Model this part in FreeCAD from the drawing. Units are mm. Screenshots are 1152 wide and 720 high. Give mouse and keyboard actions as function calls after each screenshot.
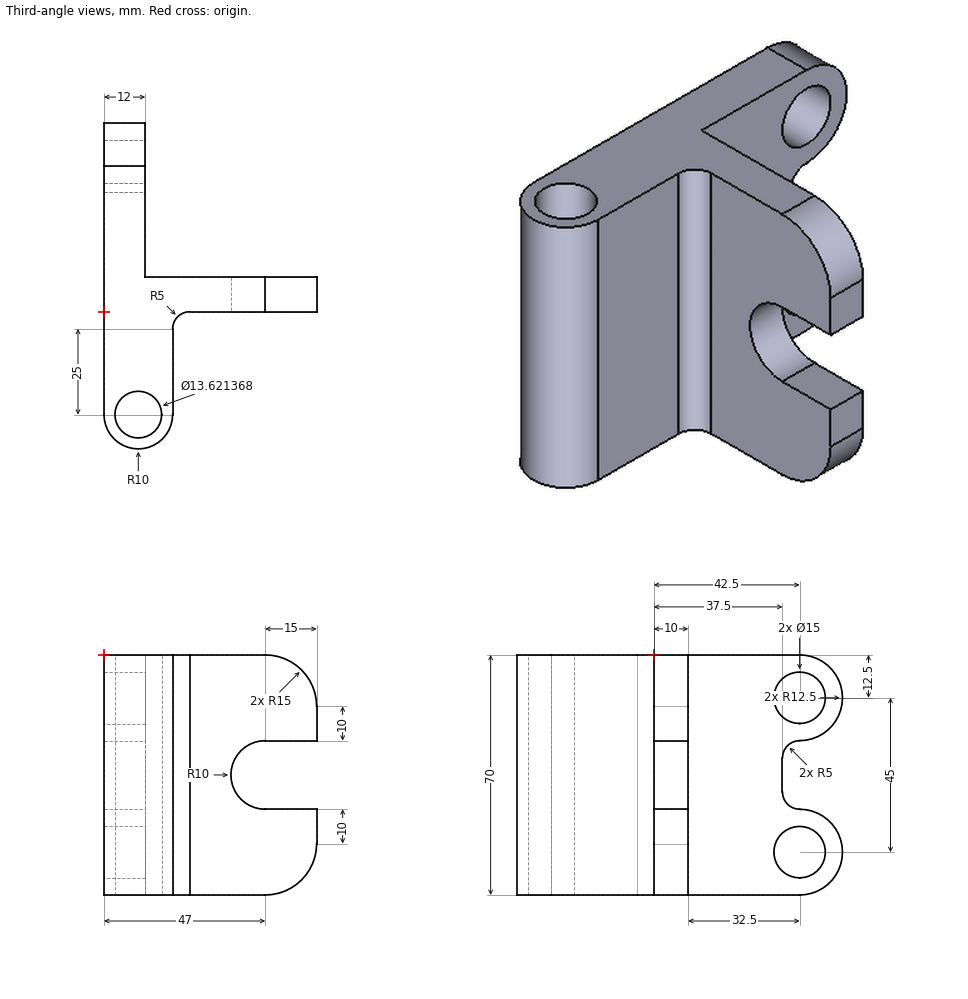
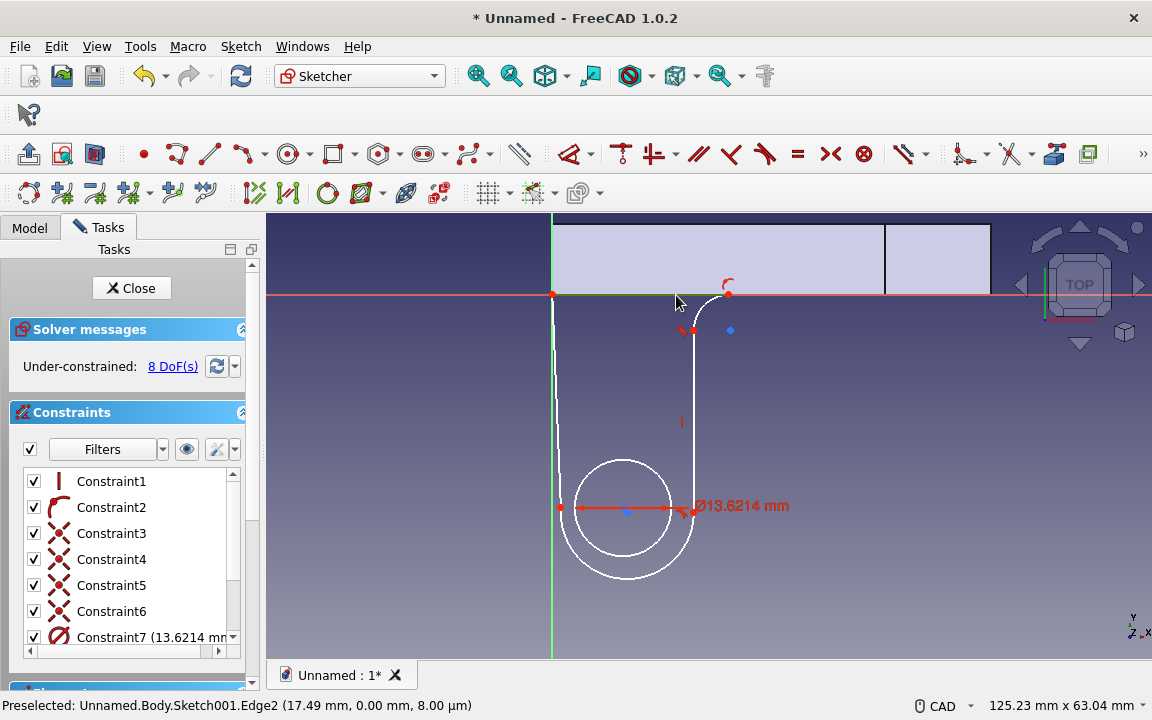
click(698, 315)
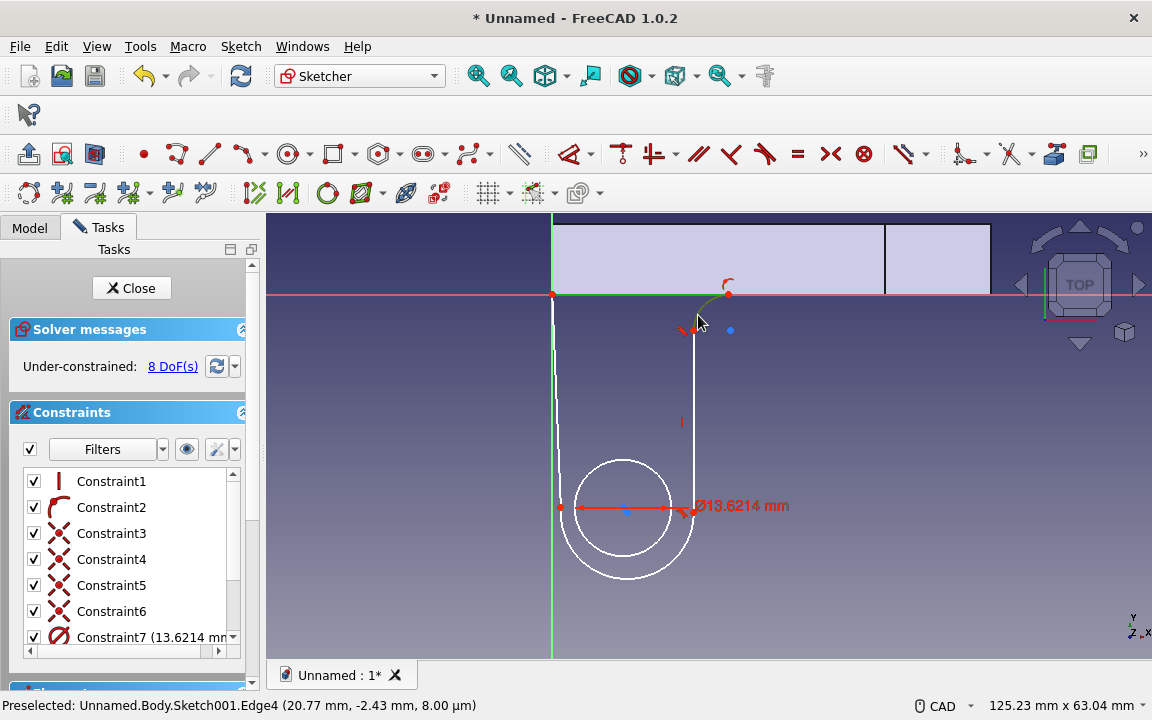
click(765, 154)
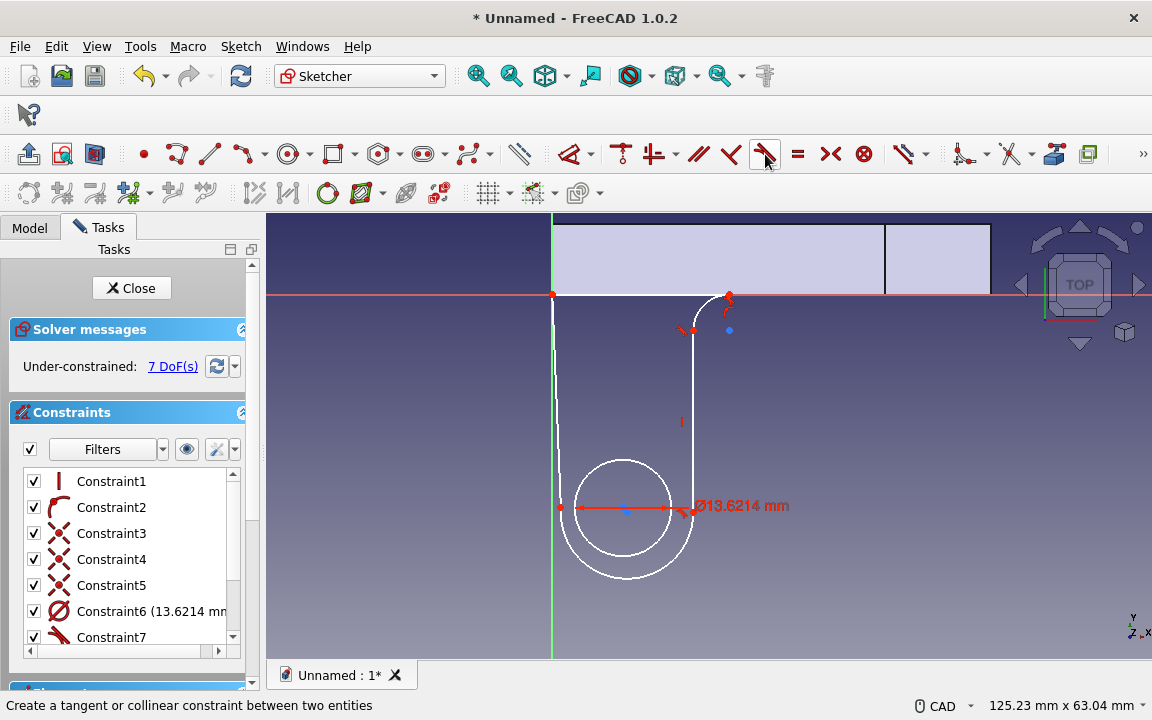
click(555, 359)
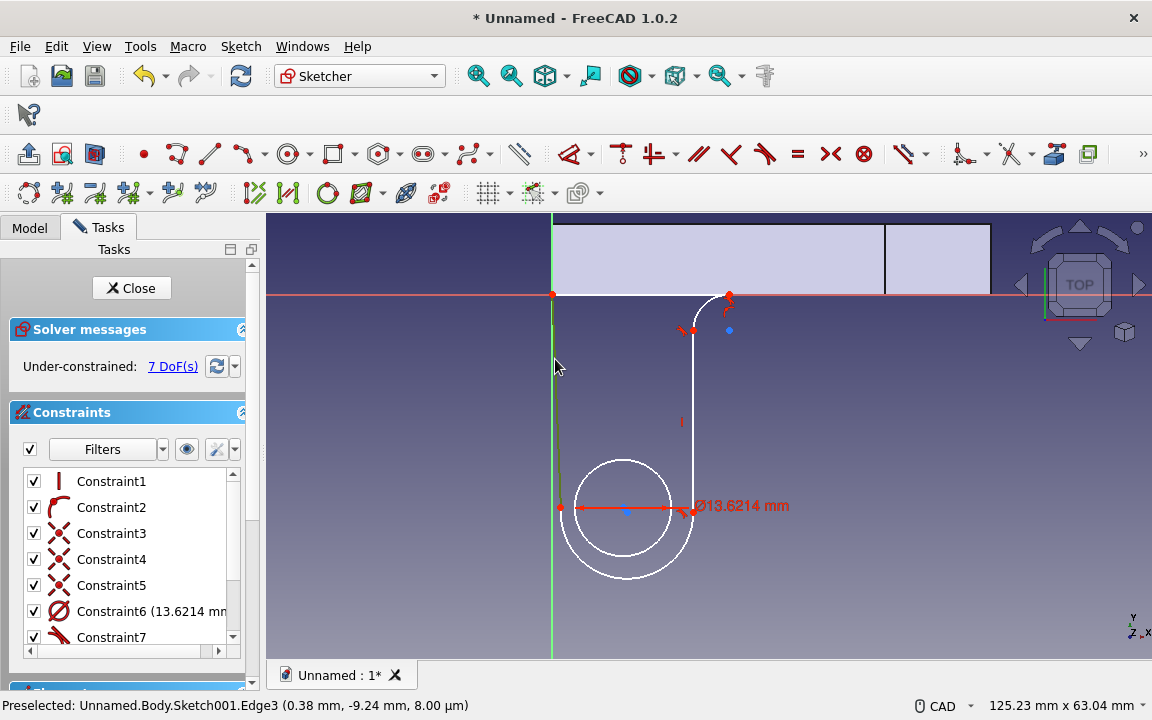
click(586, 564)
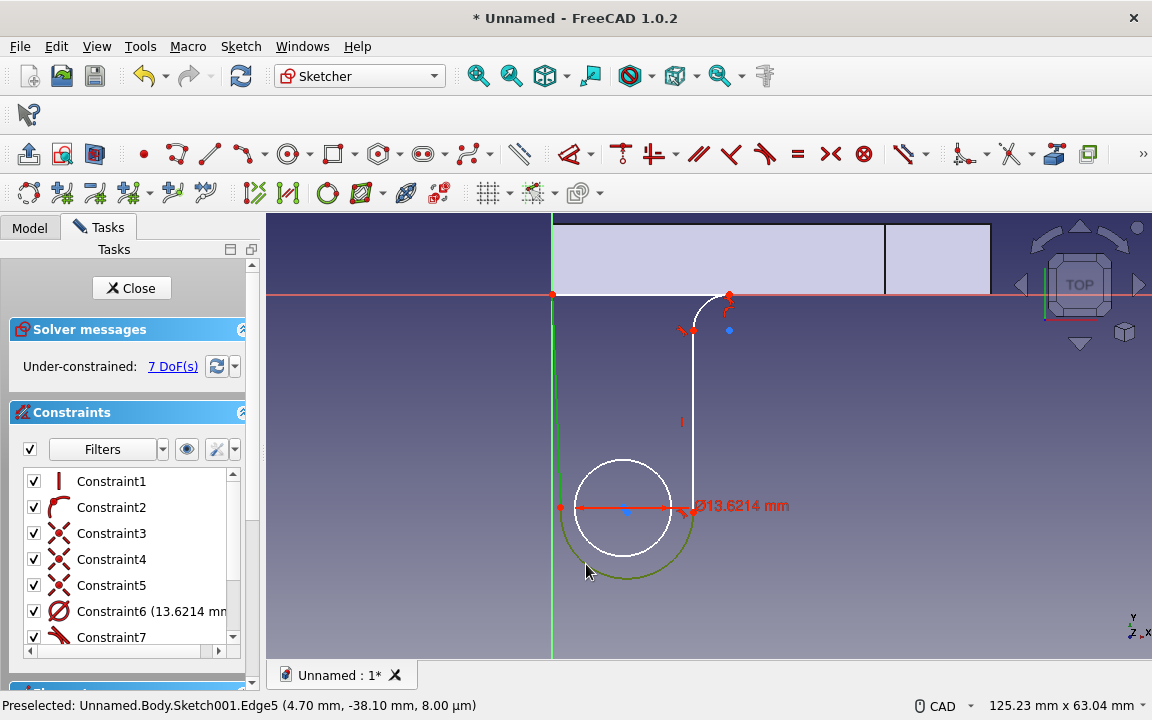
key(t)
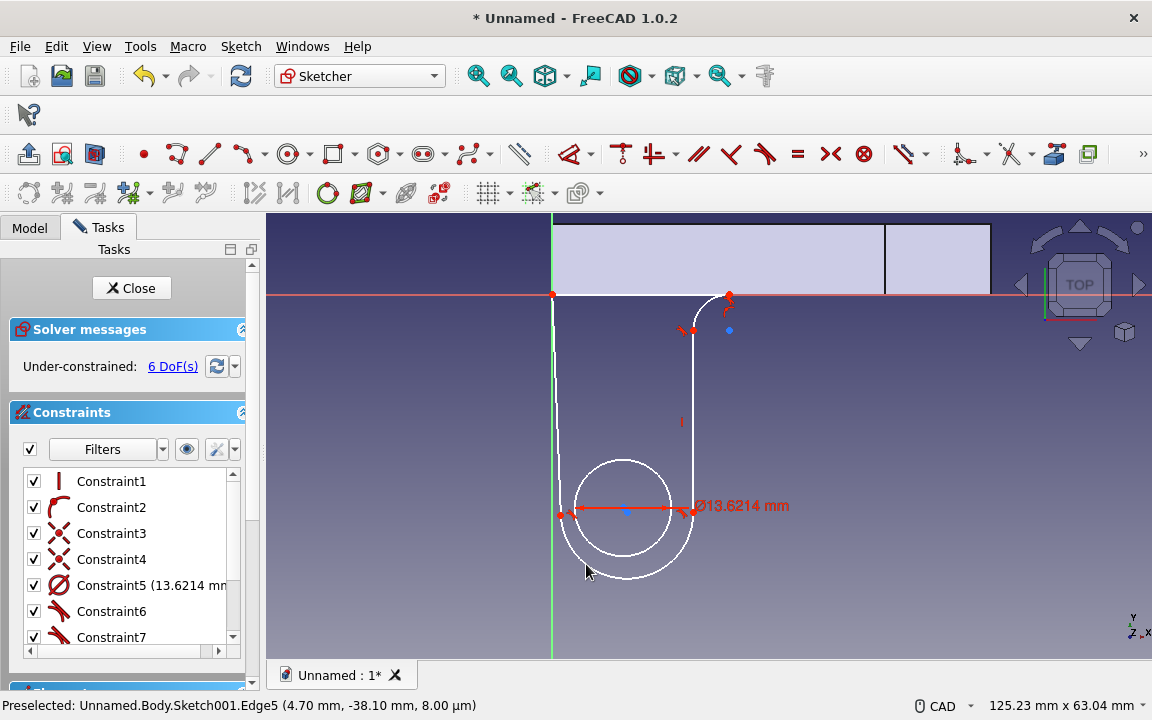
click(555, 361)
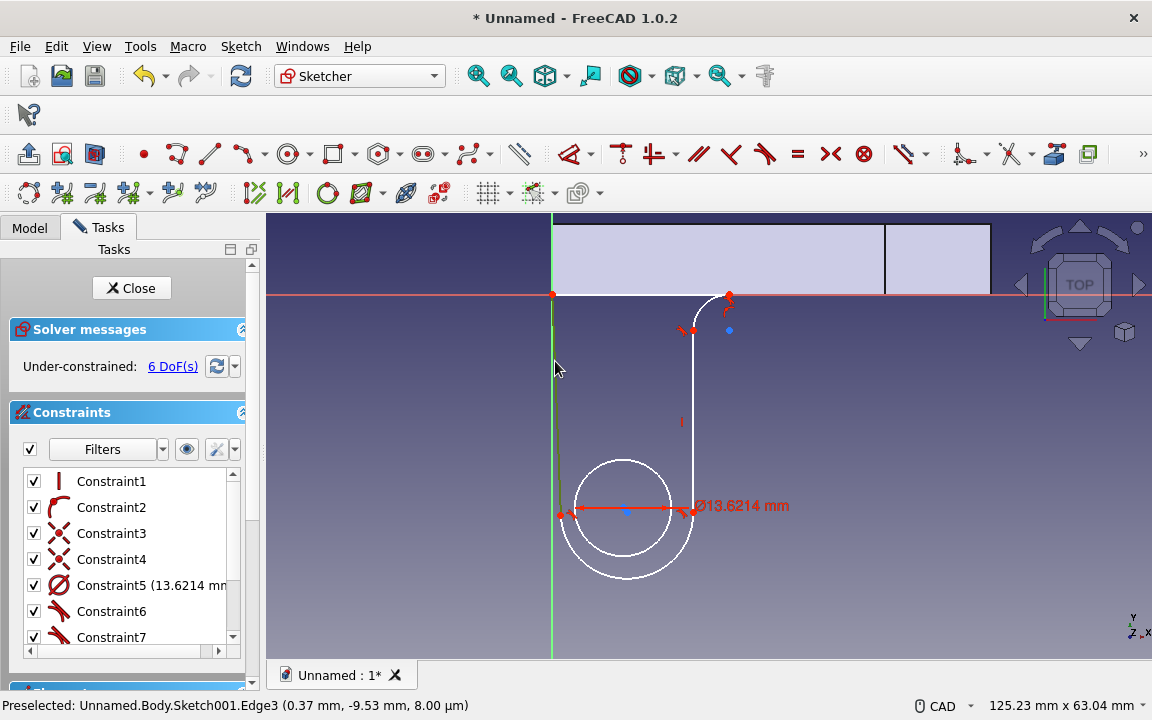
key(v)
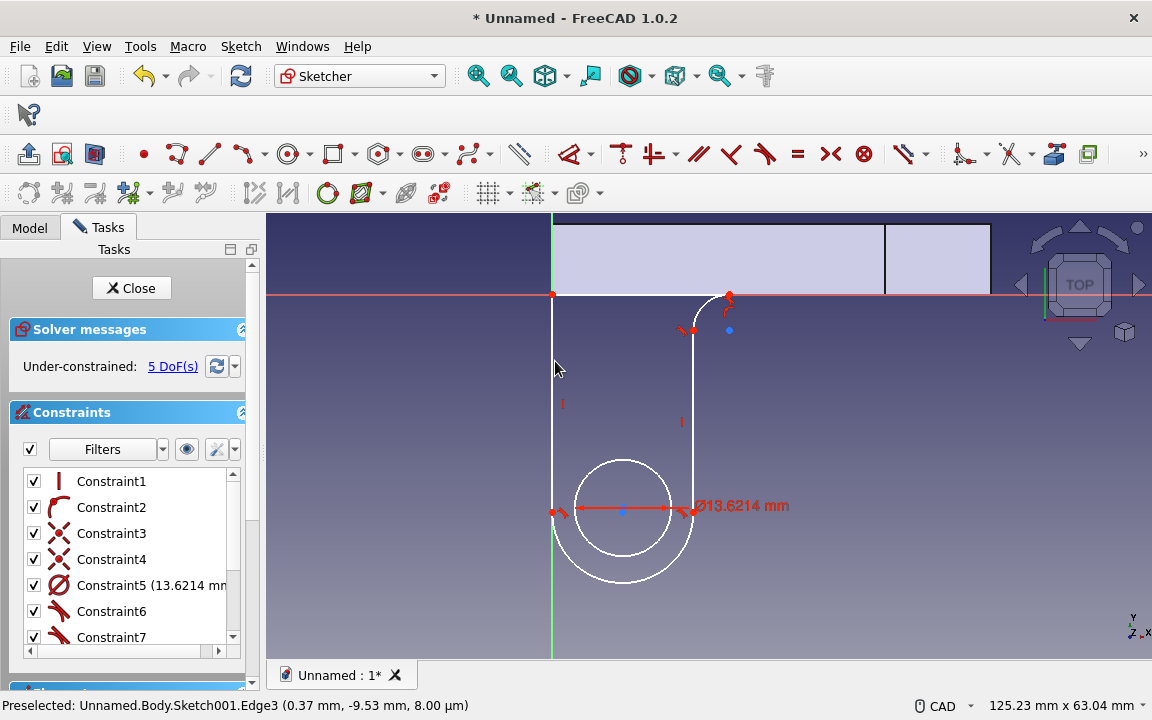
click(657, 474)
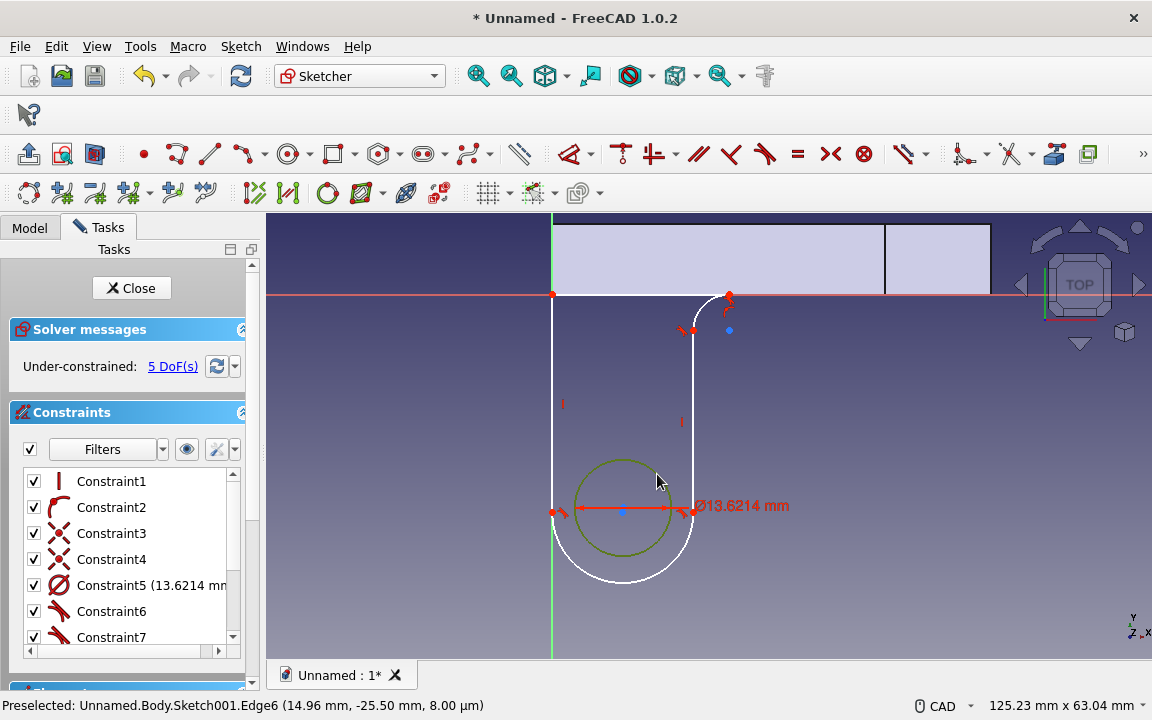
click(581, 570)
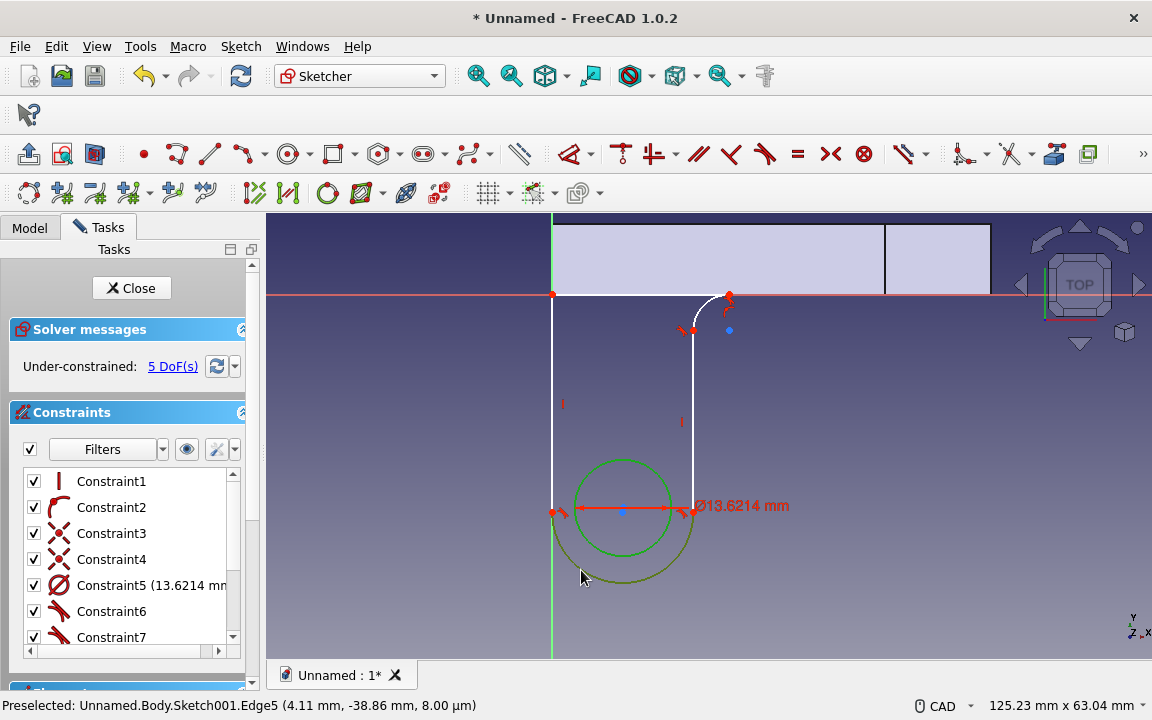
click(621, 154)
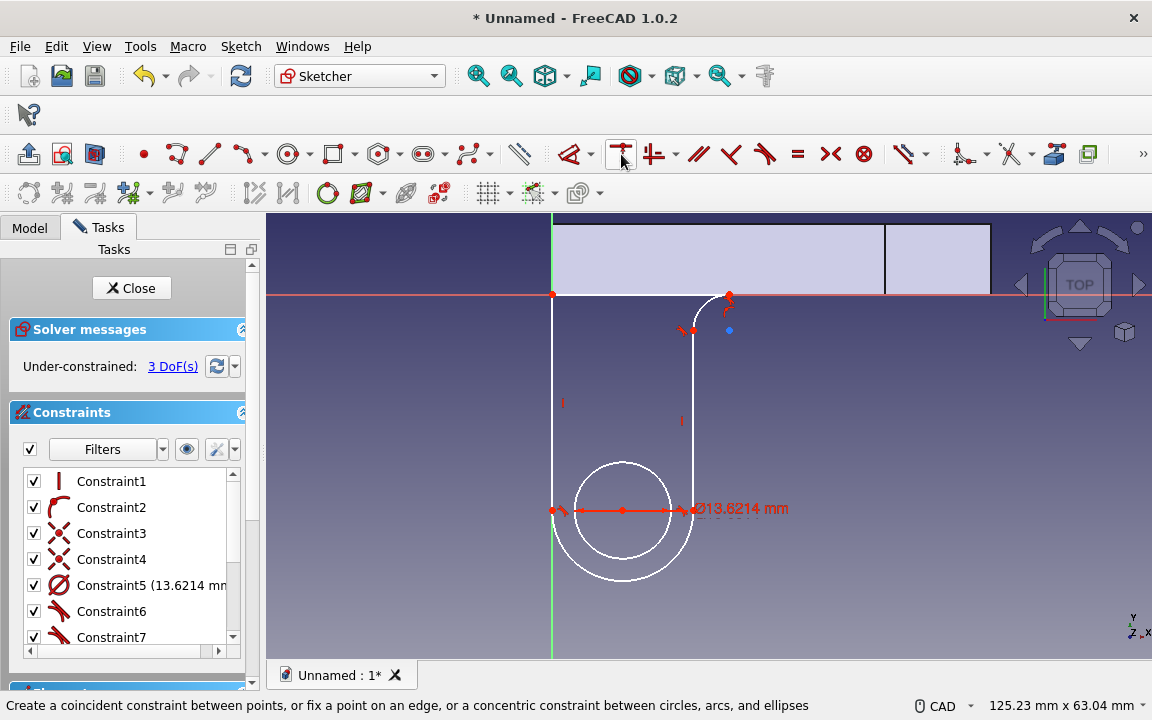
click(568, 154)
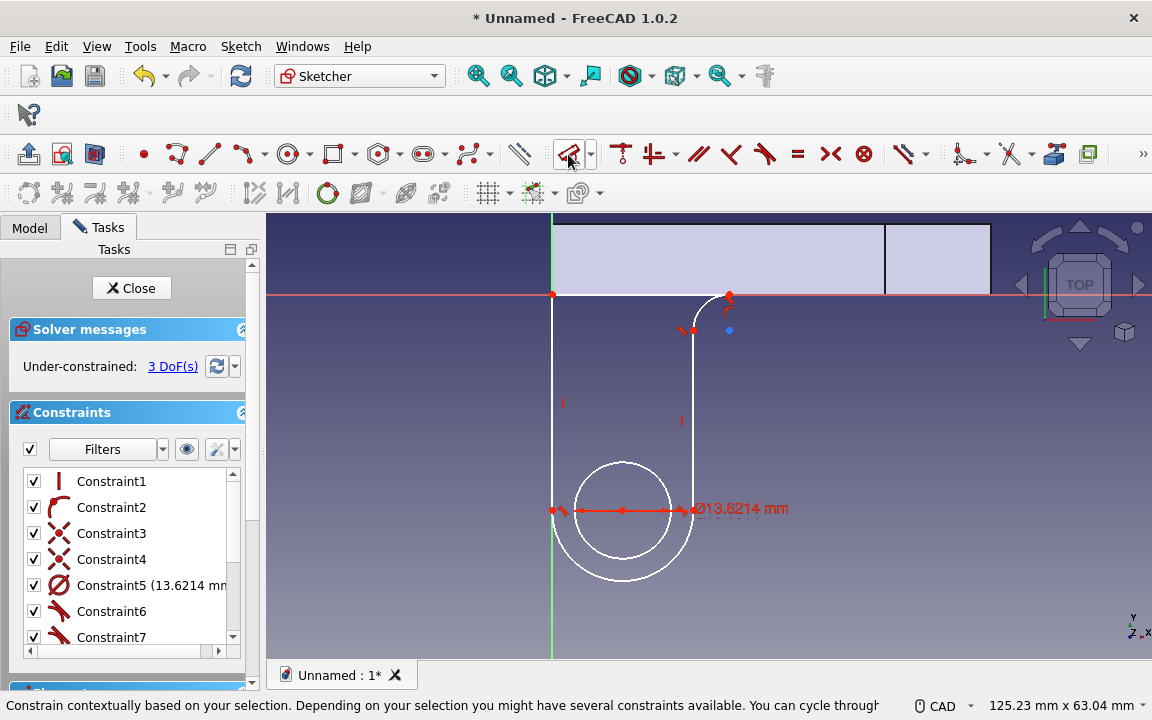
click(697, 314)
click(691, 274)